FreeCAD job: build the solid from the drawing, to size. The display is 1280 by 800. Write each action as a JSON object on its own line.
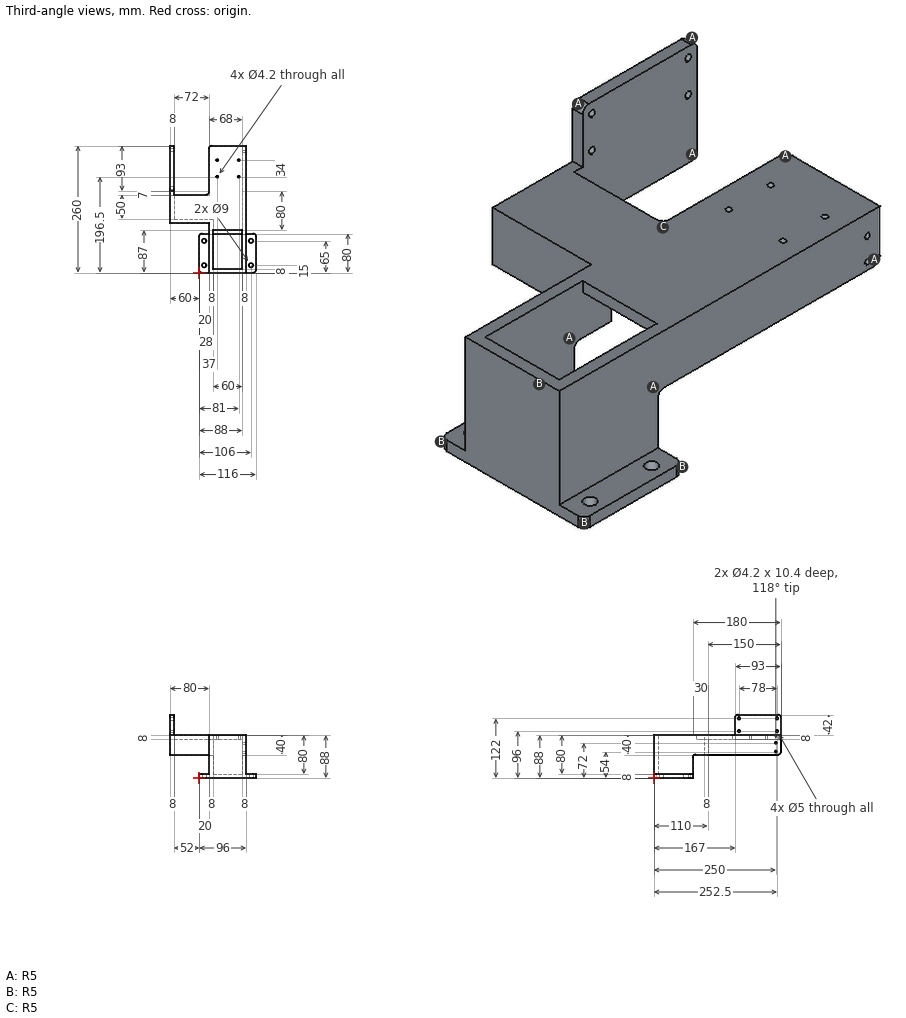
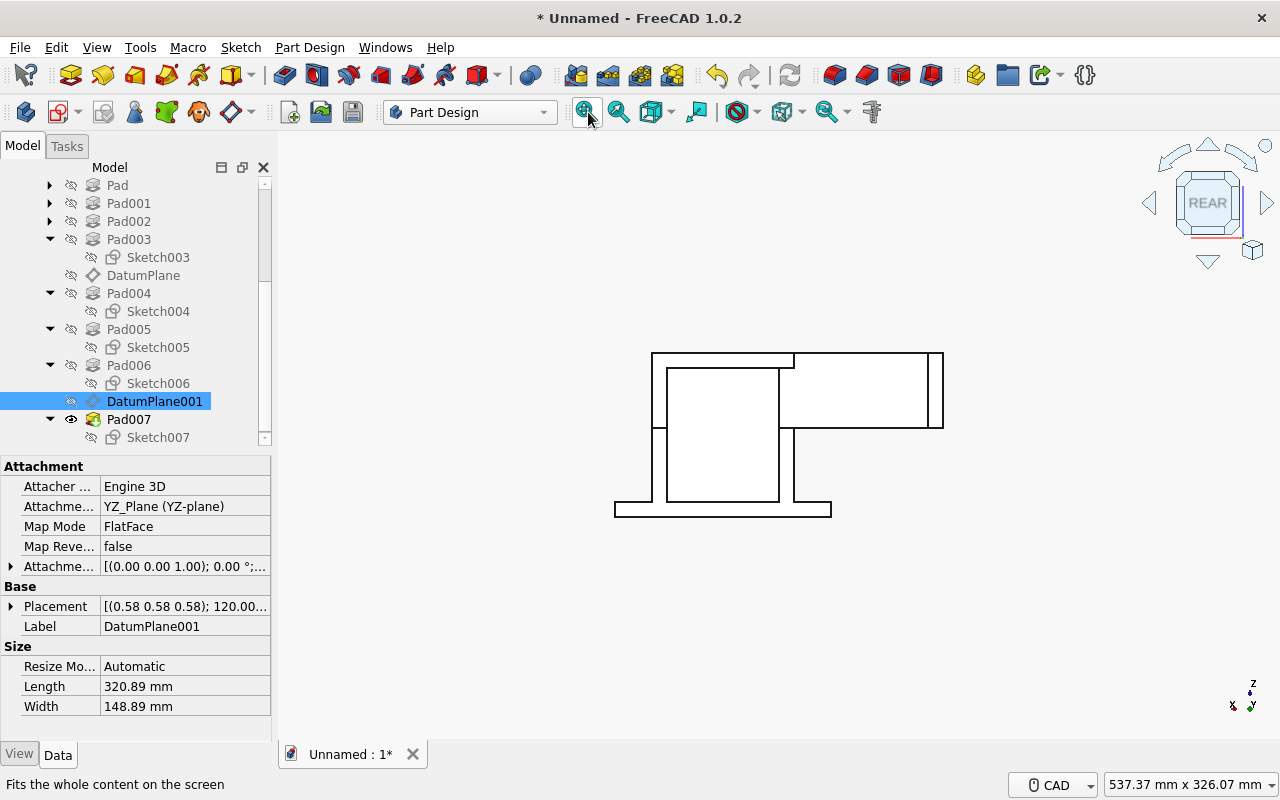
{"action": "key", "text": "0"}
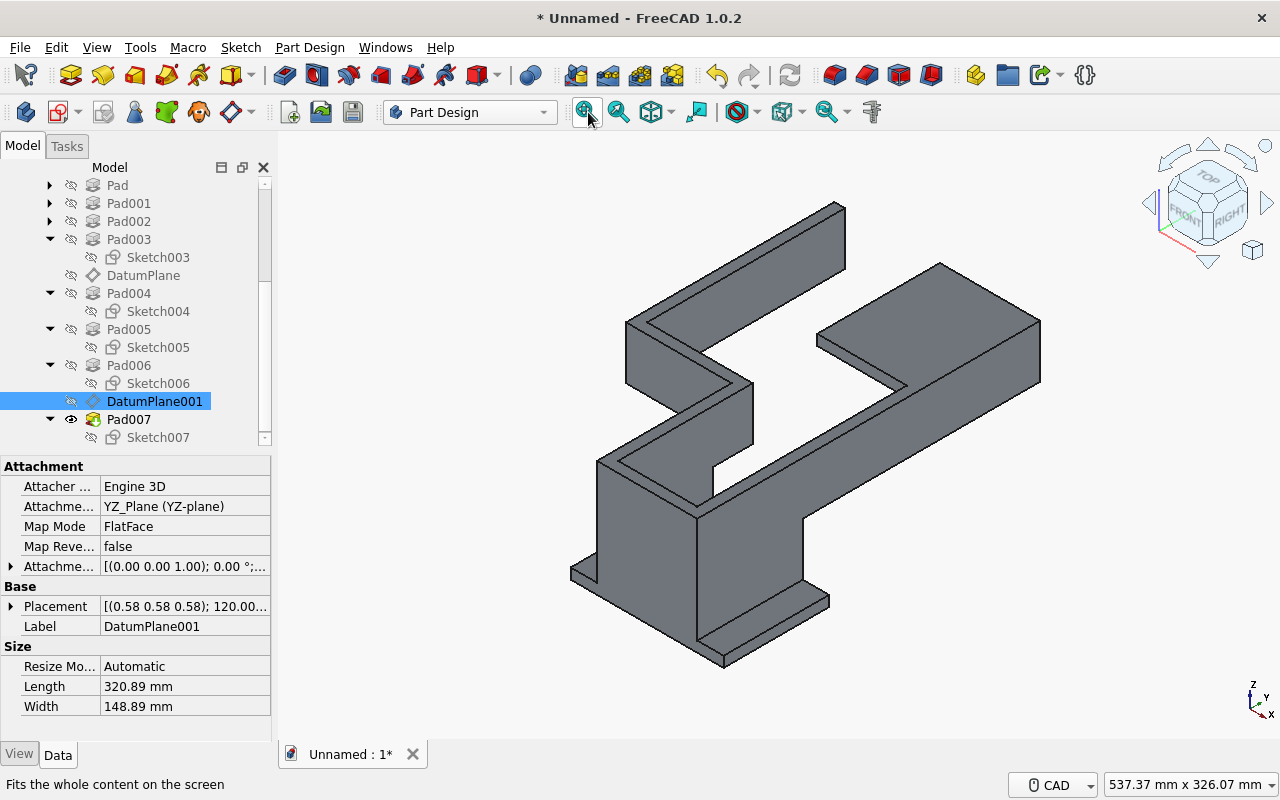
{"action": "left_click", "coordinate": [923, 337]}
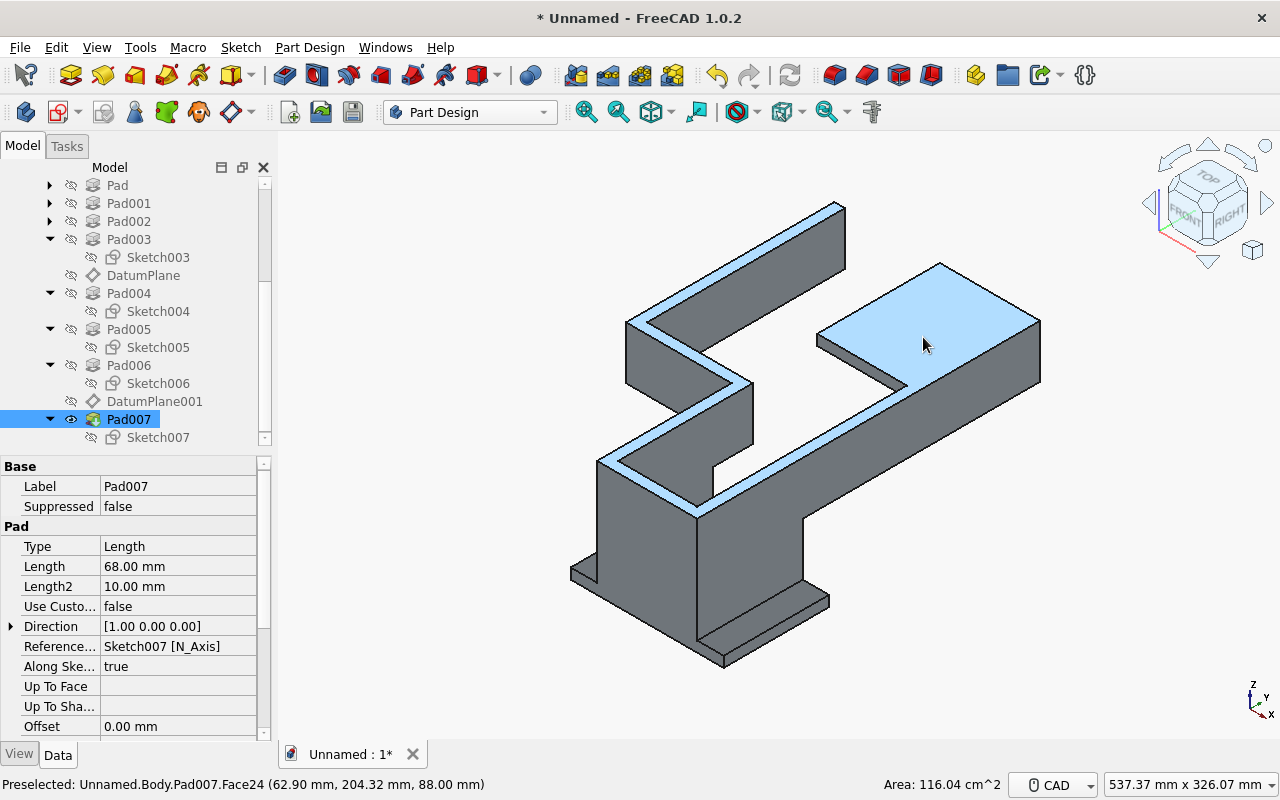
{"action": "left_click", "coordinate": [58, 112]}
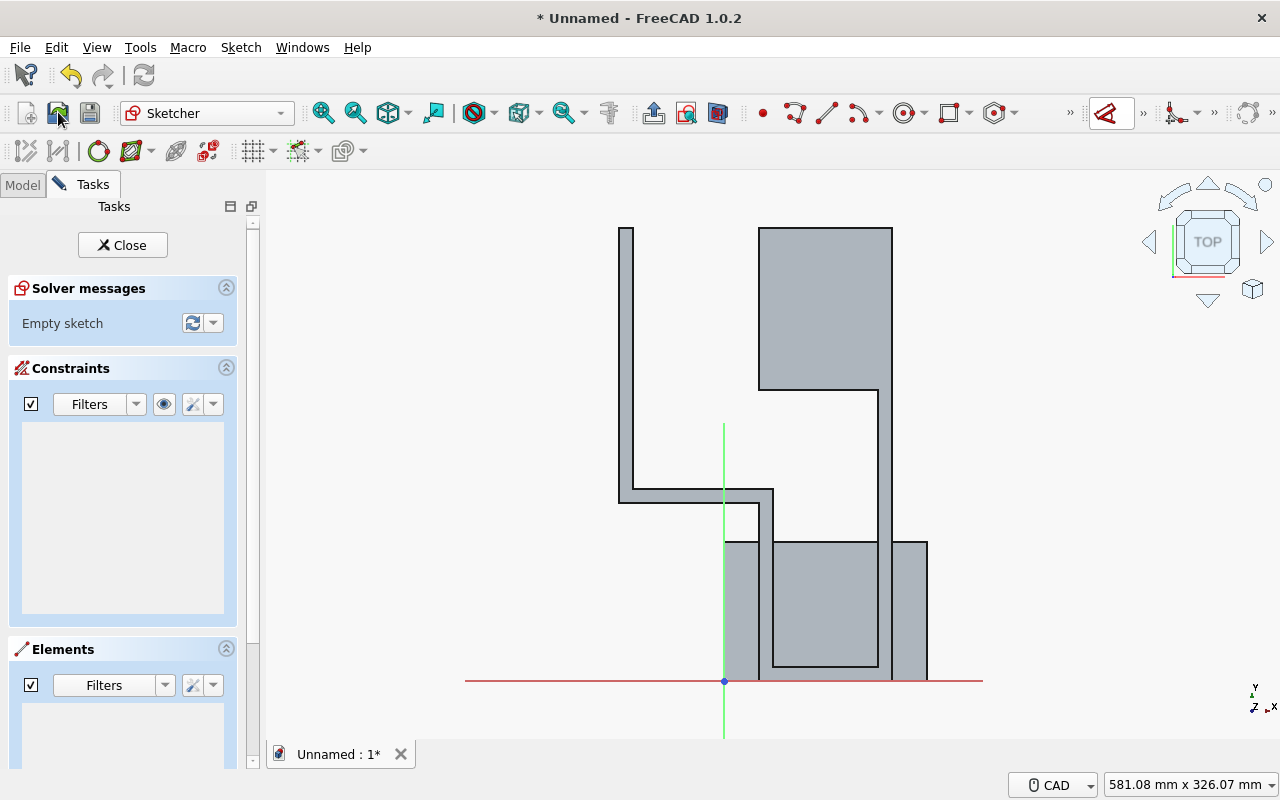
{"action": "scroll", "coordinate": [563, 198], "scroll_direction": "up", "scroll_amount": 4}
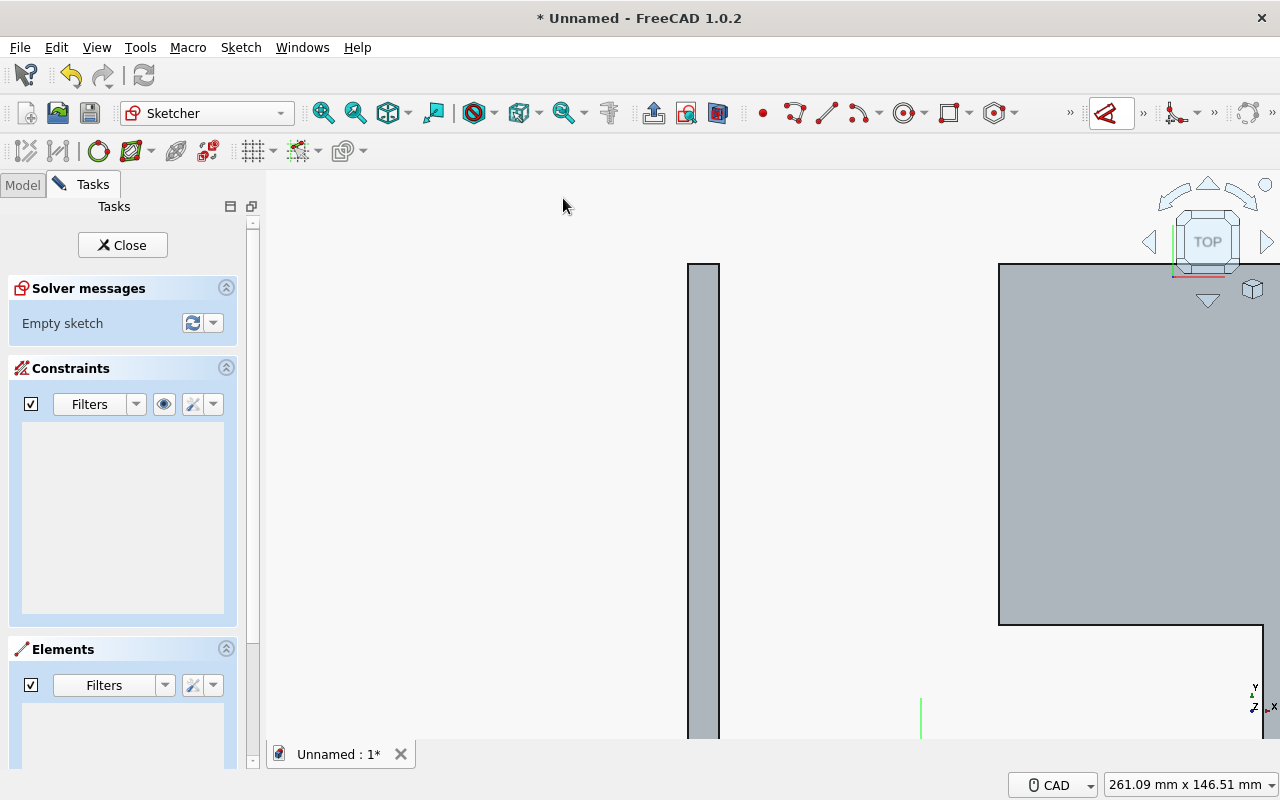
{"action": "left_click", "coordinate": [950, 114]}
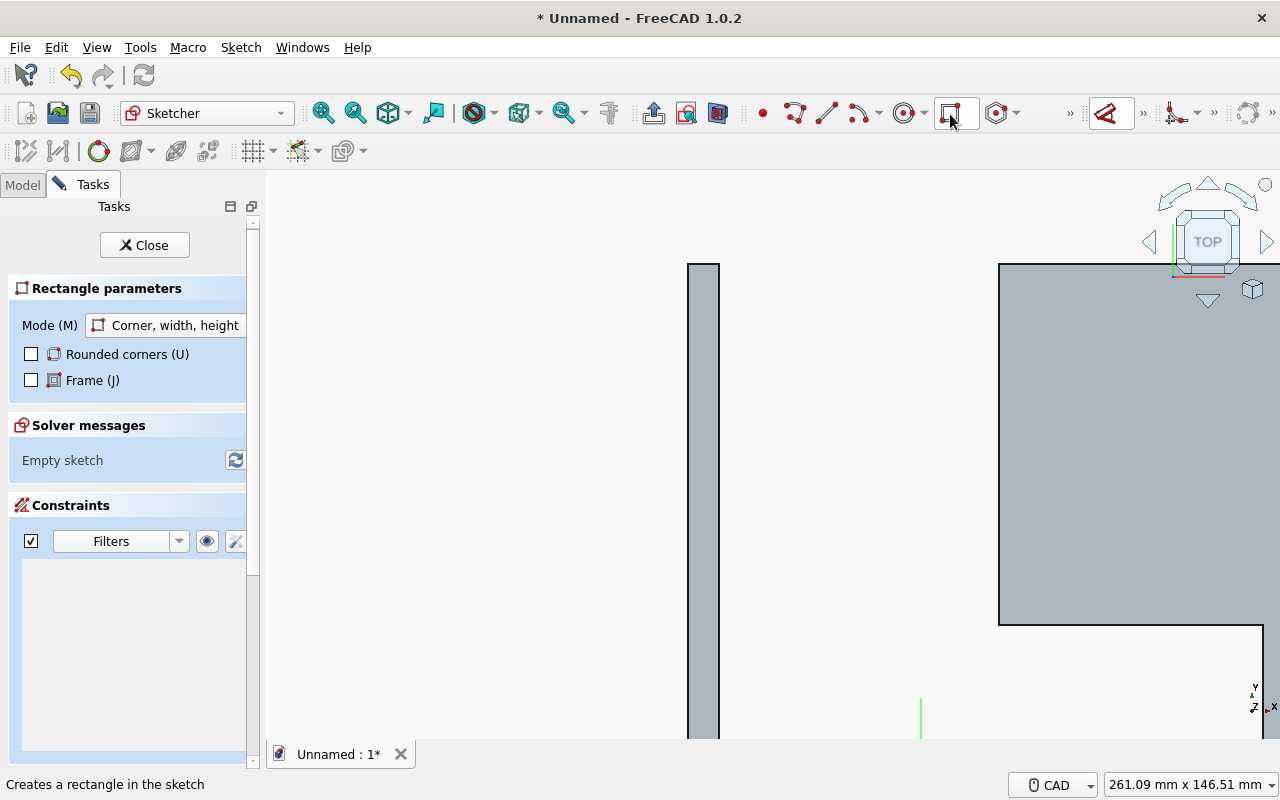
{"action": "left_click", "coordinate": [688, 264]}
{"action": "left_click", "coordinate": [719, 625]}
{"action": "key", "text": "Escape"}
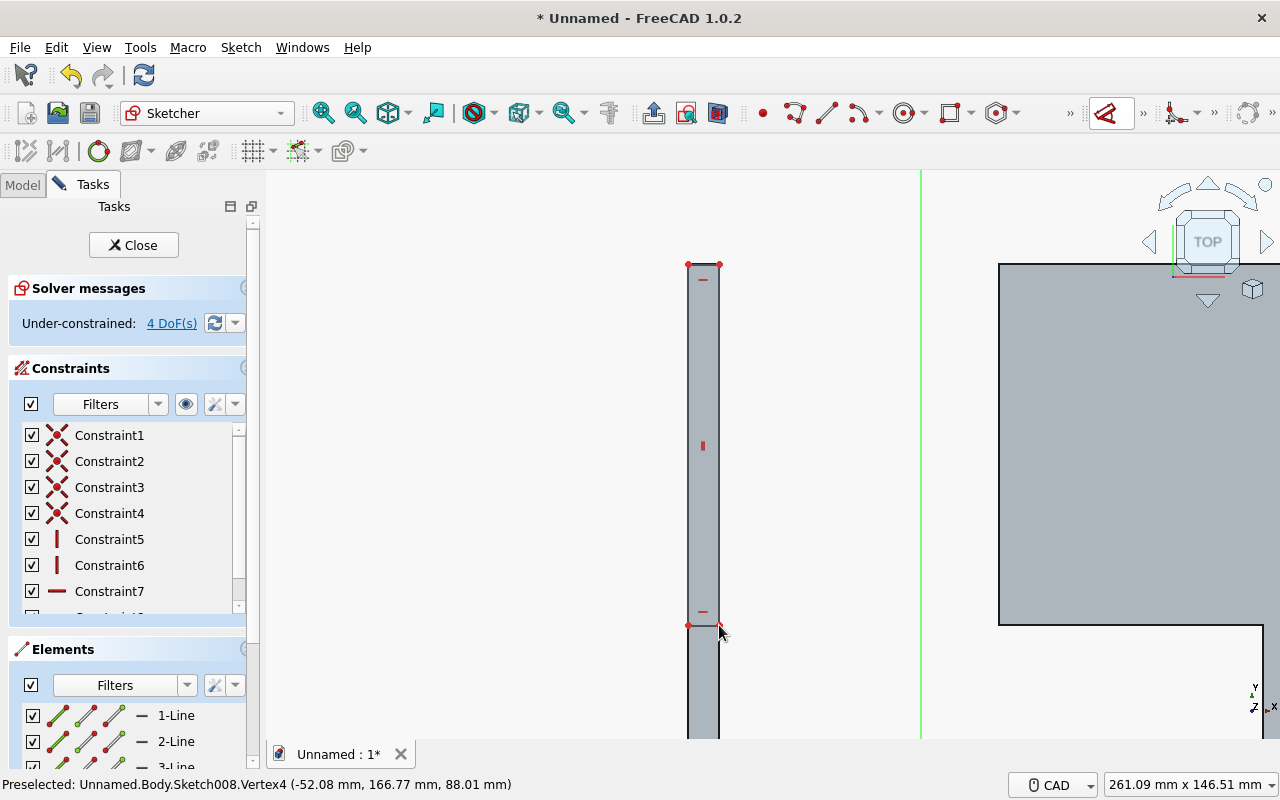
{"action": "scroll", "coordinate": [697, 626], "scroll_direction": "up", "scroll_amount": 2}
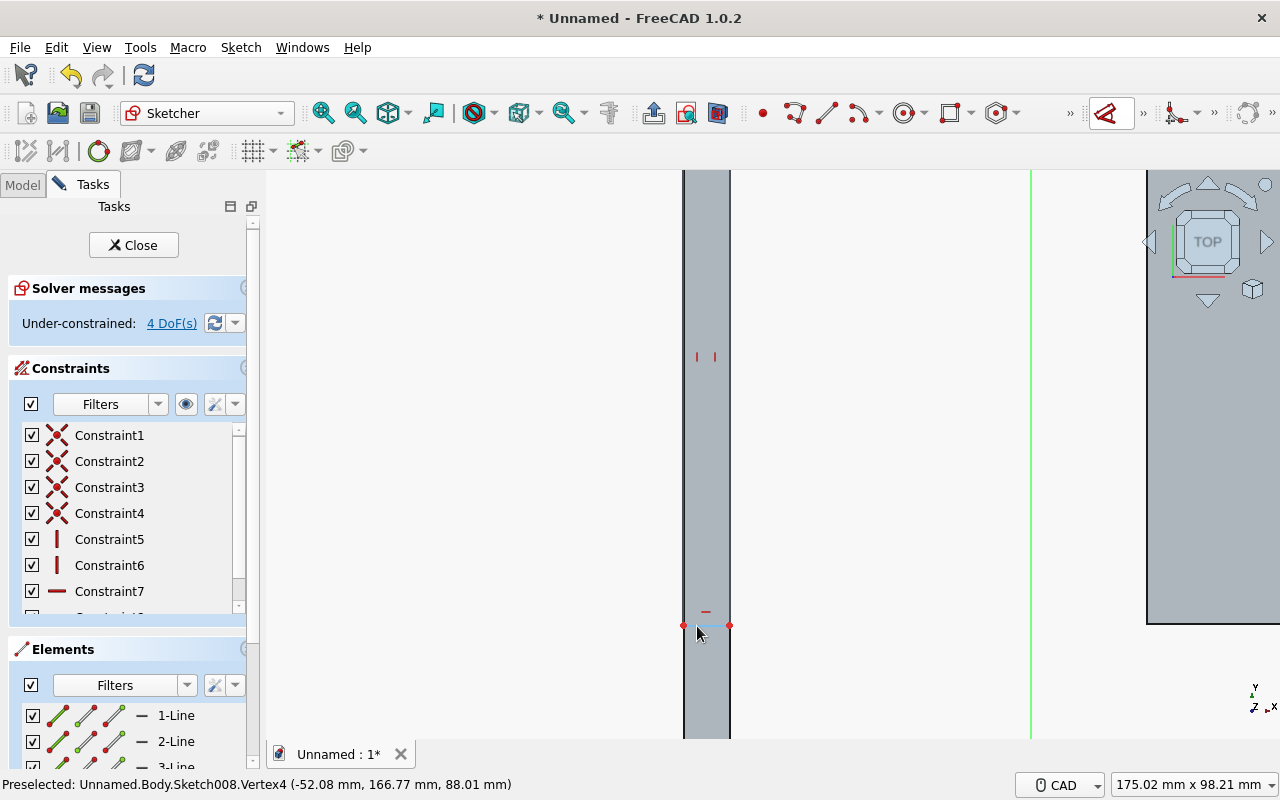
{"action": "left_click", "coordinate": [697, 626]}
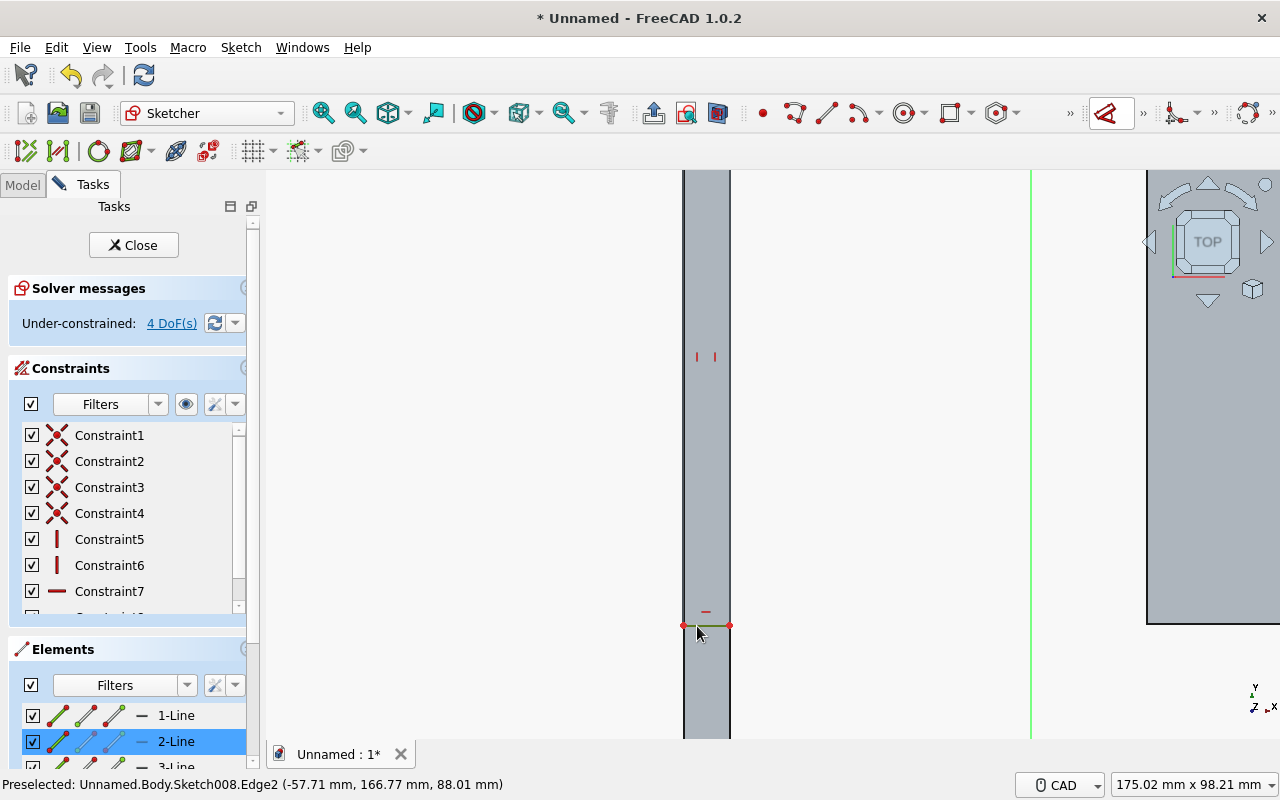
{"action": "key", "text": "l"}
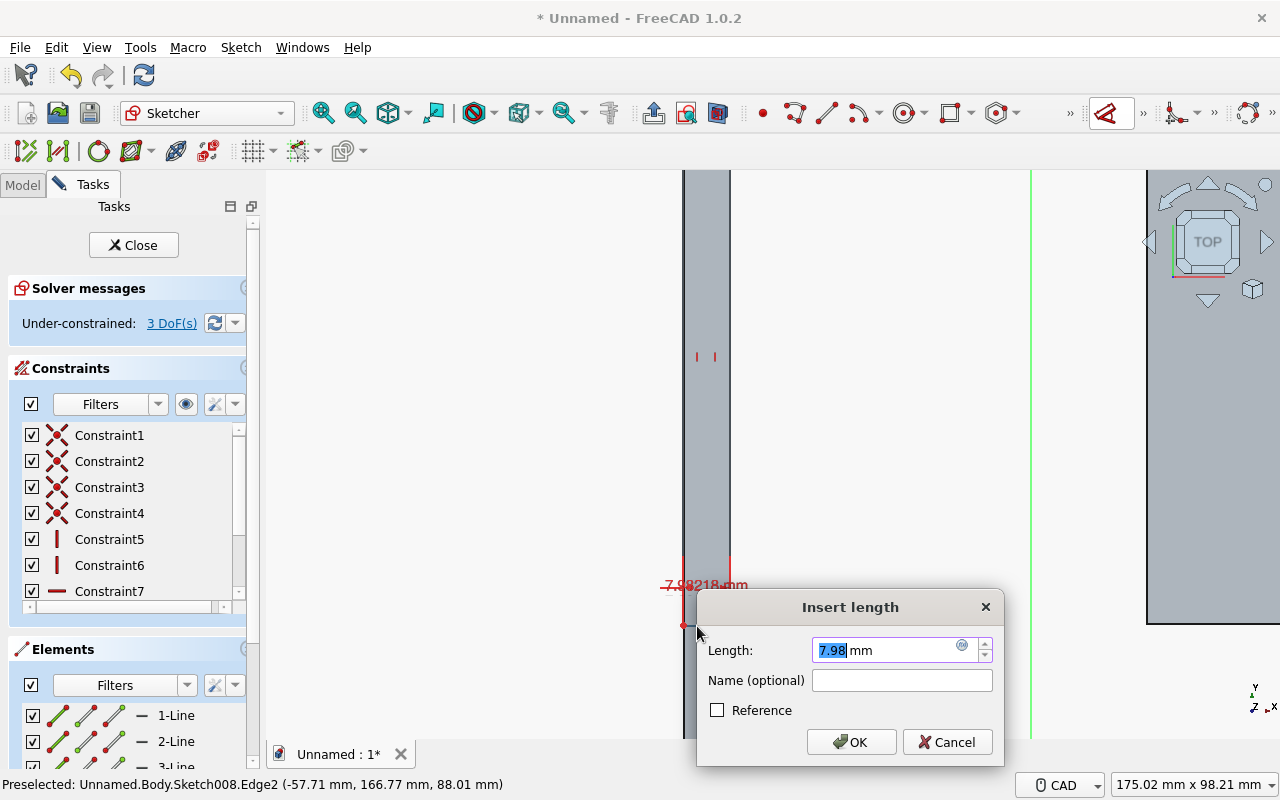
{"action": "type", "text": "8"}
{"action": "key", "text": "Return"}